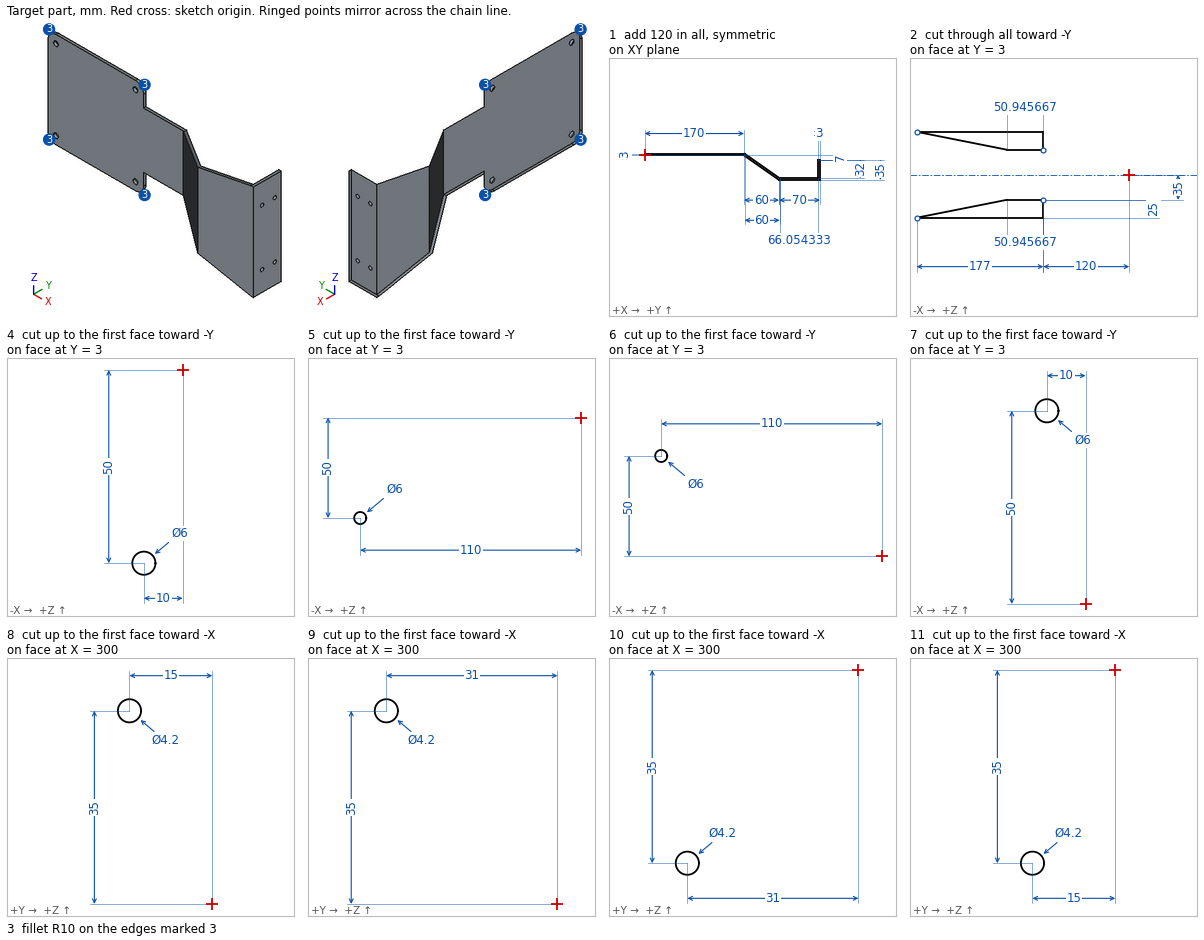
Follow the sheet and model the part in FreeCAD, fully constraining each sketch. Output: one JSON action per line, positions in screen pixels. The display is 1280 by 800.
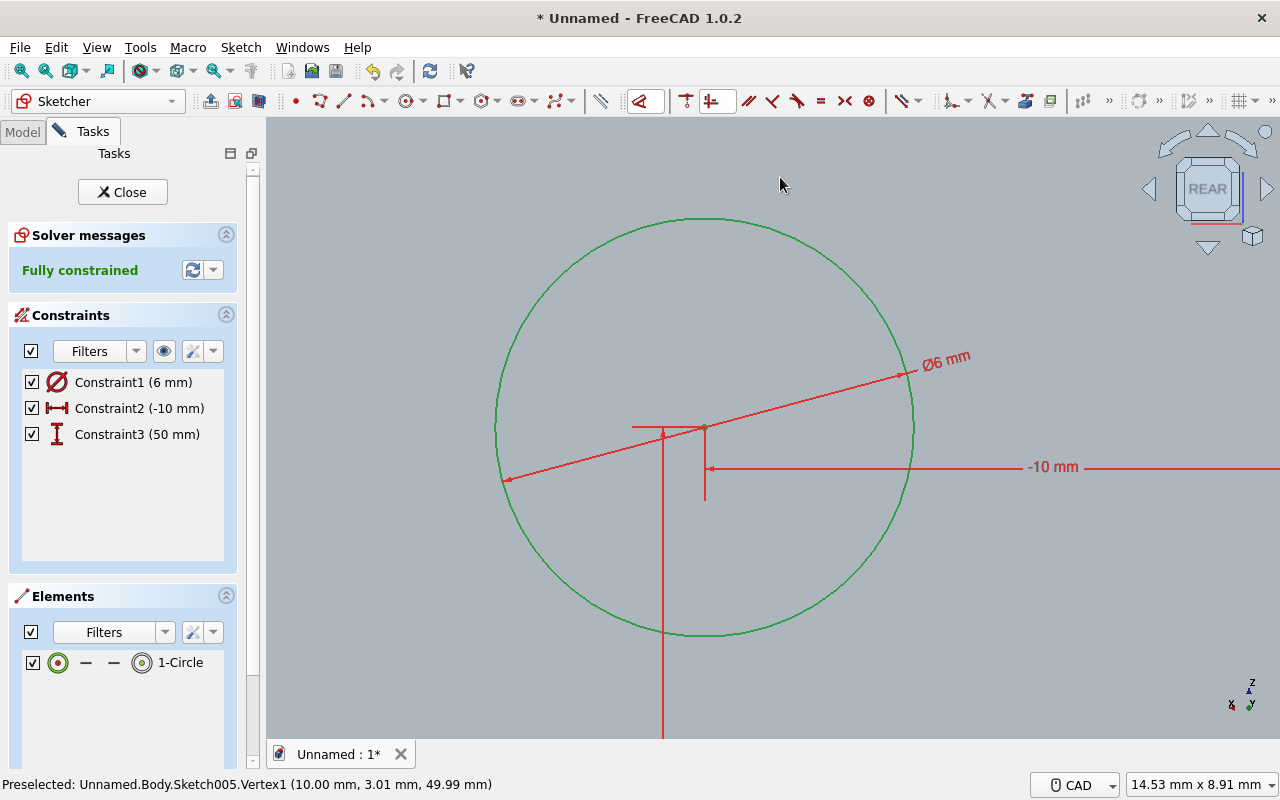
{"action": "left_click", "coordinate": [123, 192]}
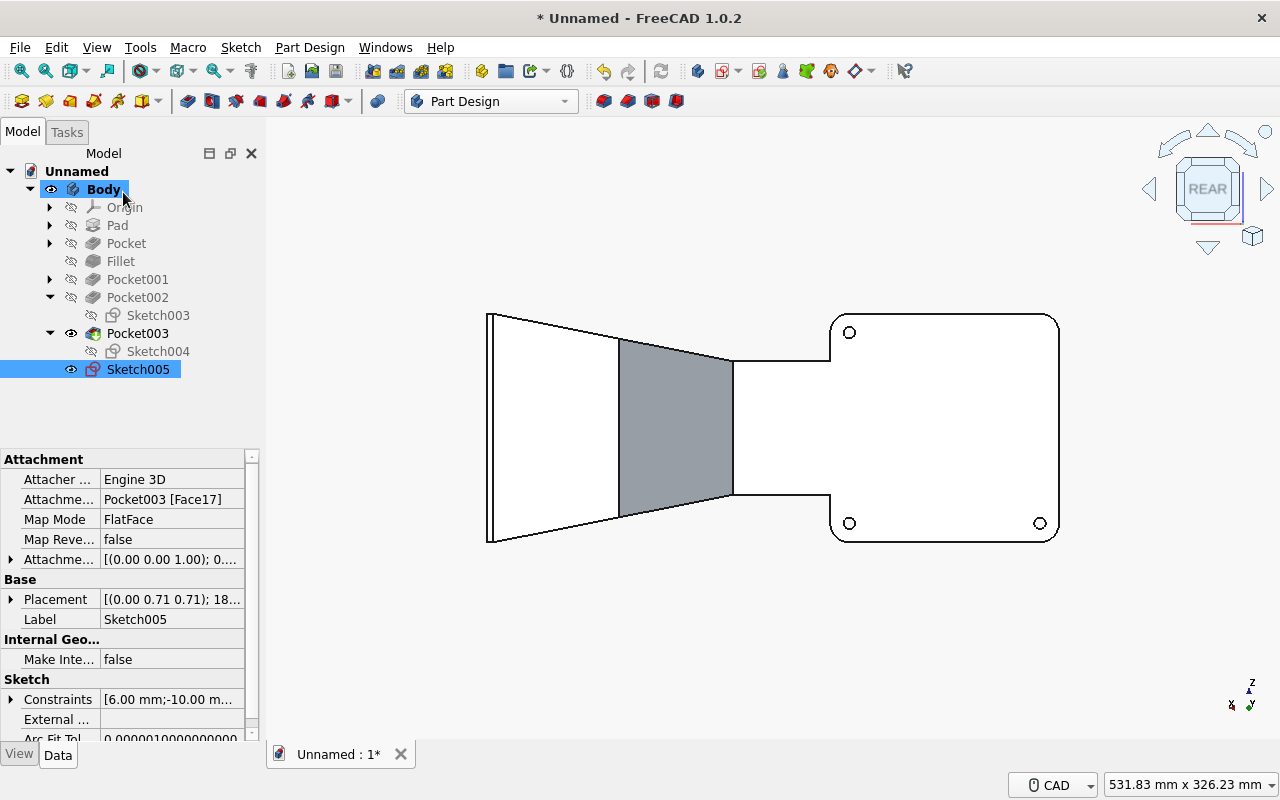
{"action": "left_click", "coordinate": [188, 102]}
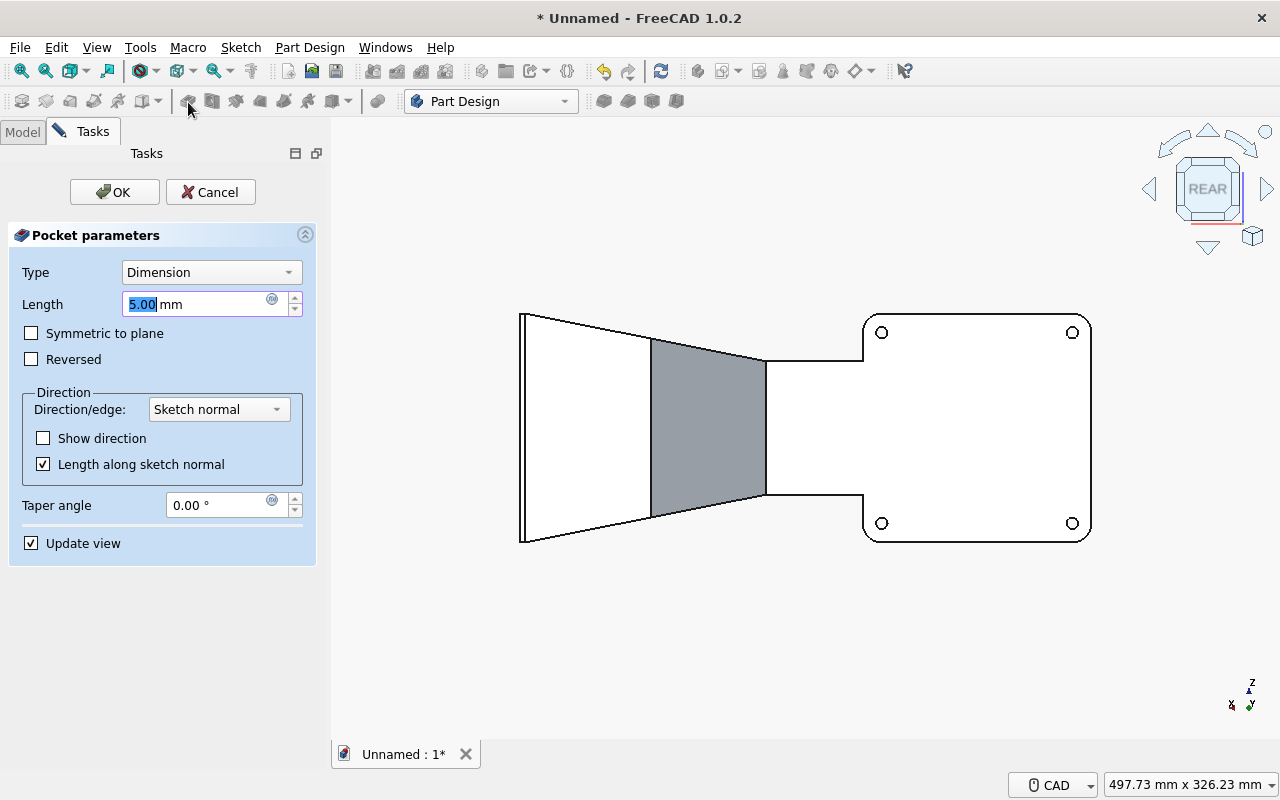
{"action": "left_click", "coordinate": [212, 272]}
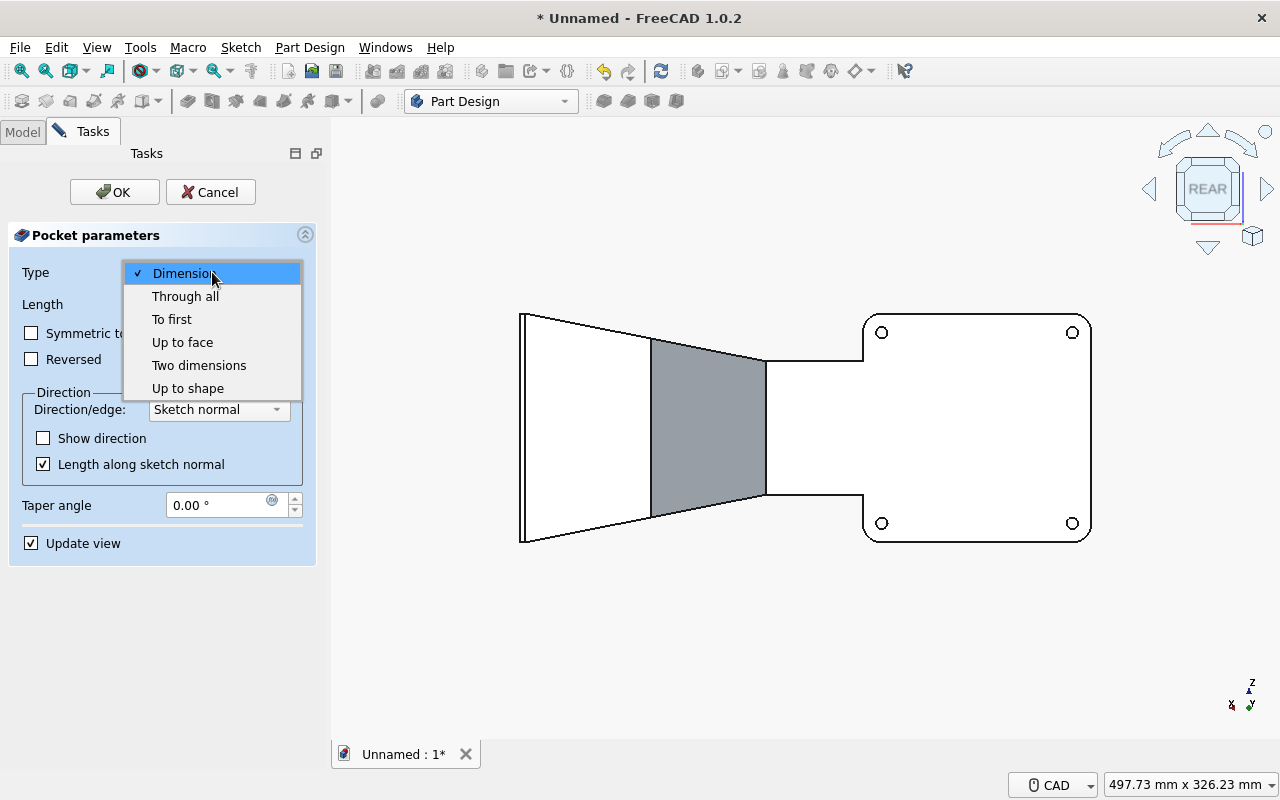
{"action": "left_click", "coordinate": [212, 320]}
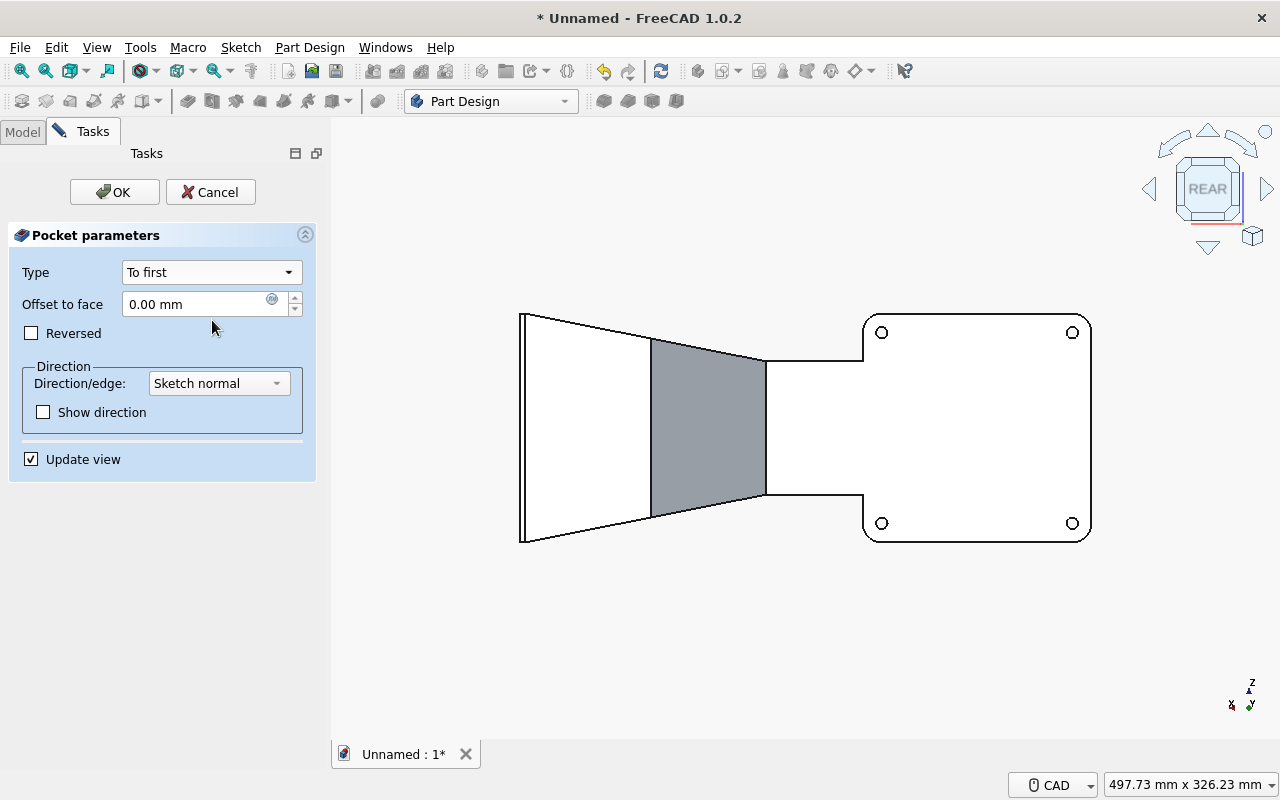
{"action": "left_click", "coordinate": [115, 192]}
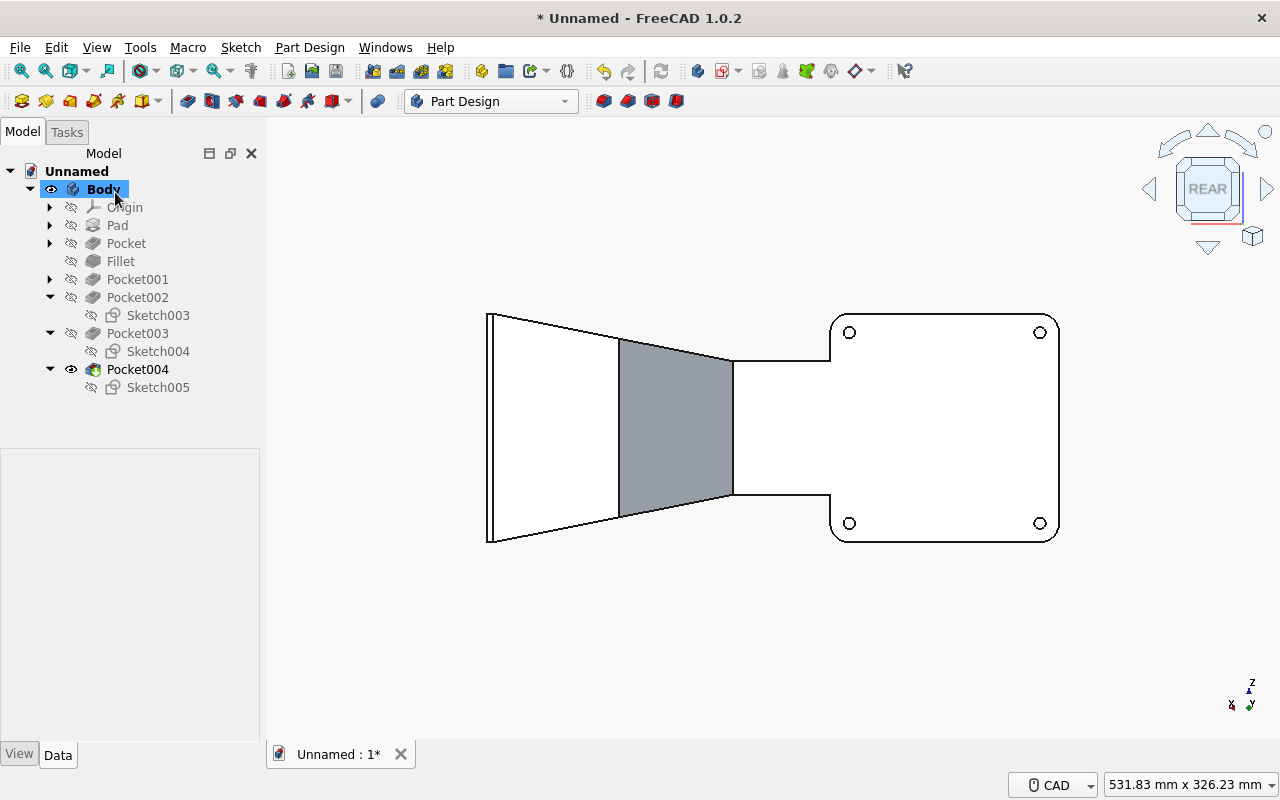
{"action": "key", "text": "0"}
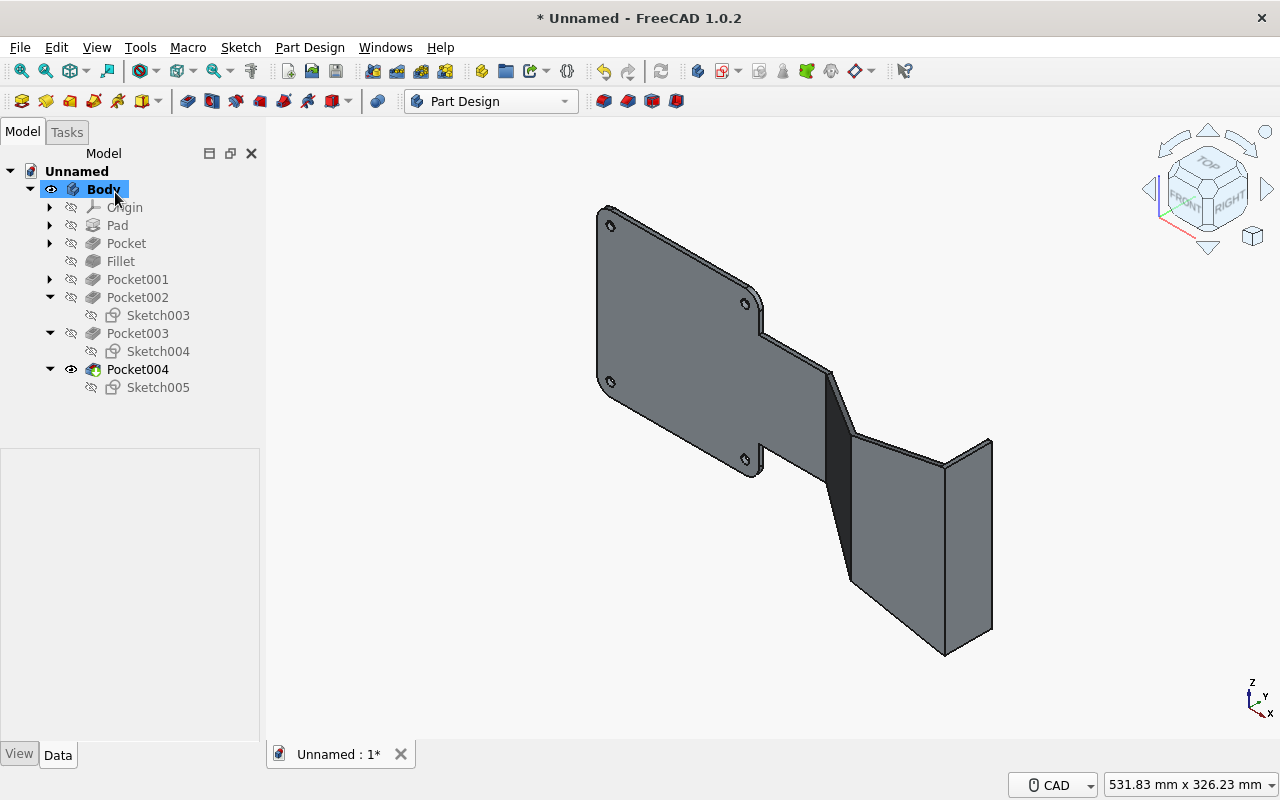
{"action": "left_click", "coordinate": [968, 494]}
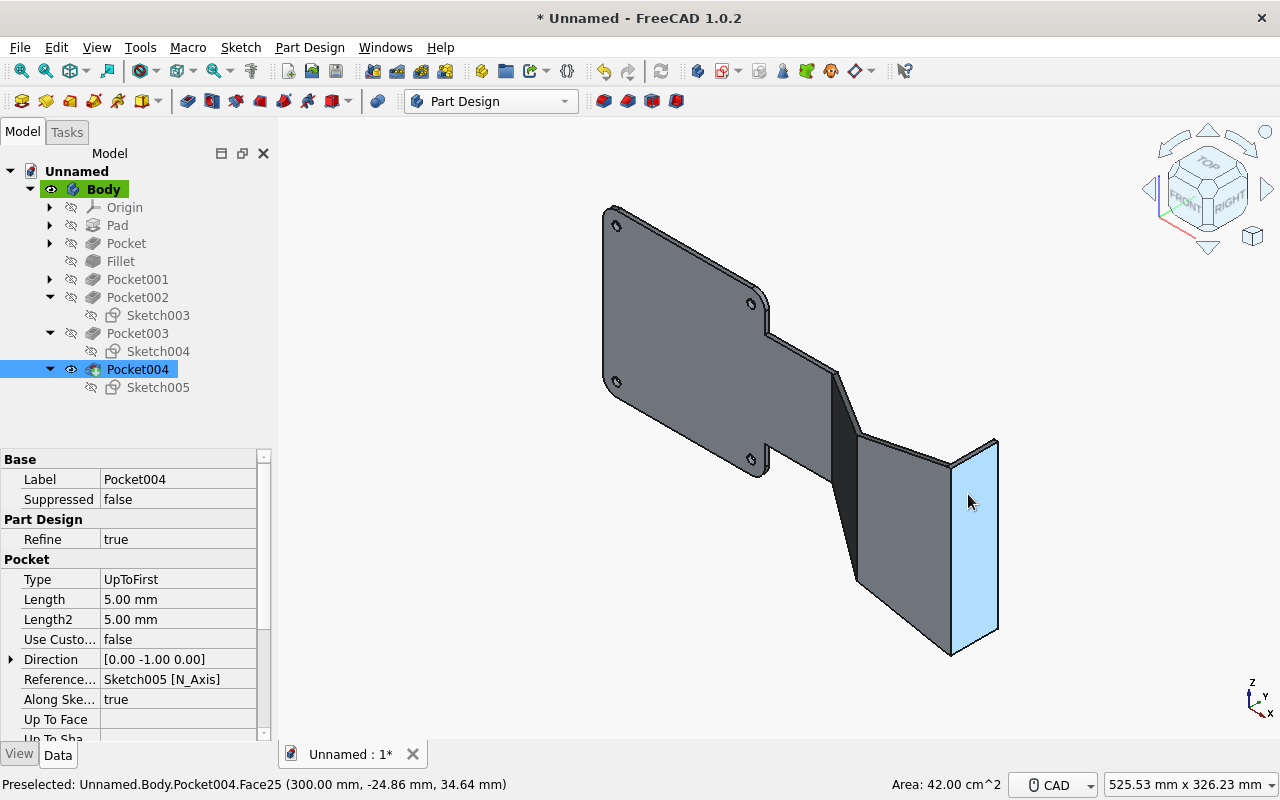
{"action": "left_click", "coordinate": [722, 72]}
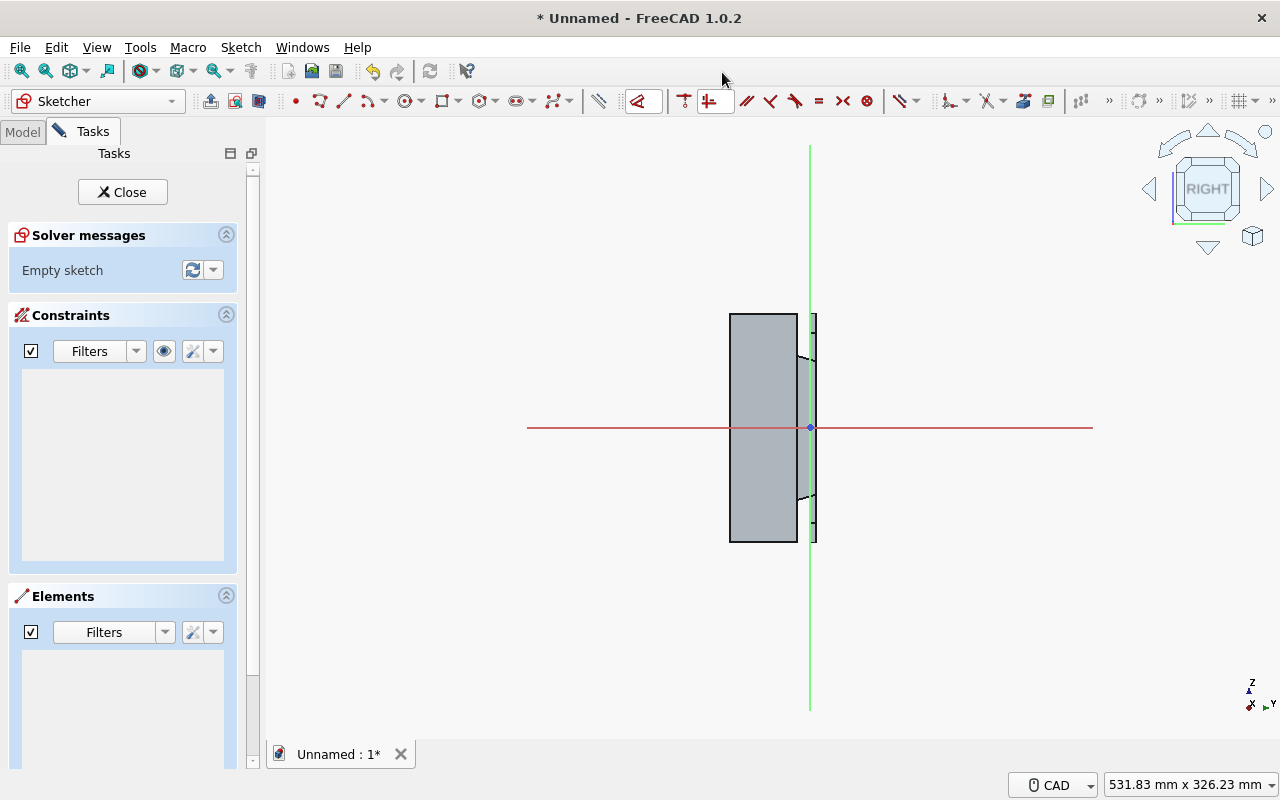
{"action": "scroll", "coordinate": [786, 358], "scroll_direction": "up", "scroll_amount": 15}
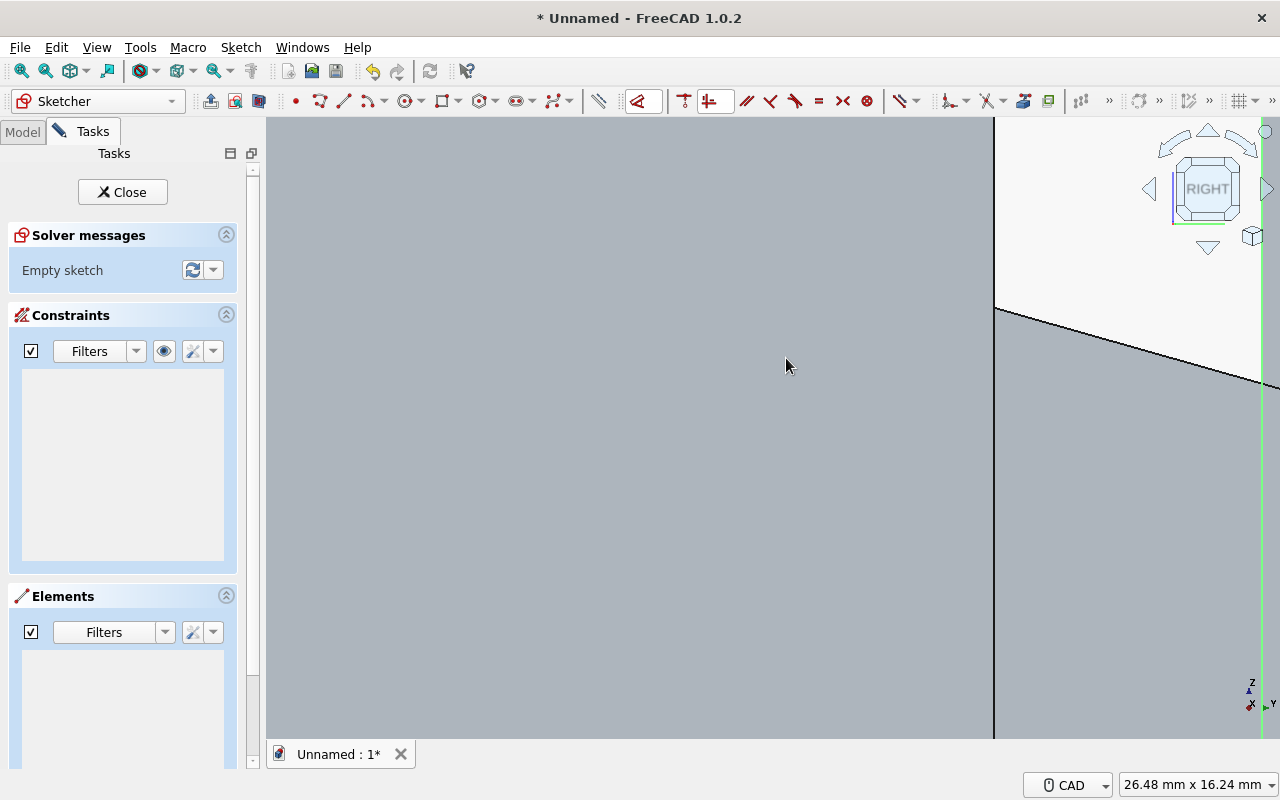
{"action": "scroll", "coordinate": [677, 409], "scroll_direction": "up", "scroll_amount": 5}